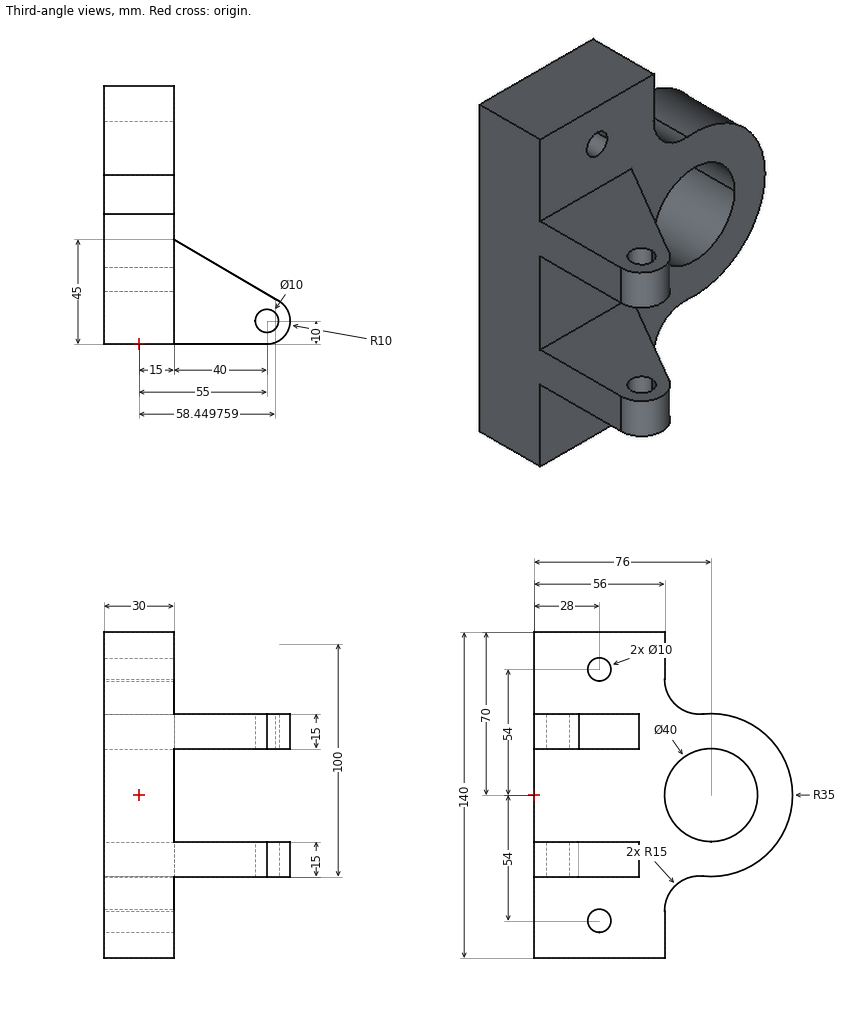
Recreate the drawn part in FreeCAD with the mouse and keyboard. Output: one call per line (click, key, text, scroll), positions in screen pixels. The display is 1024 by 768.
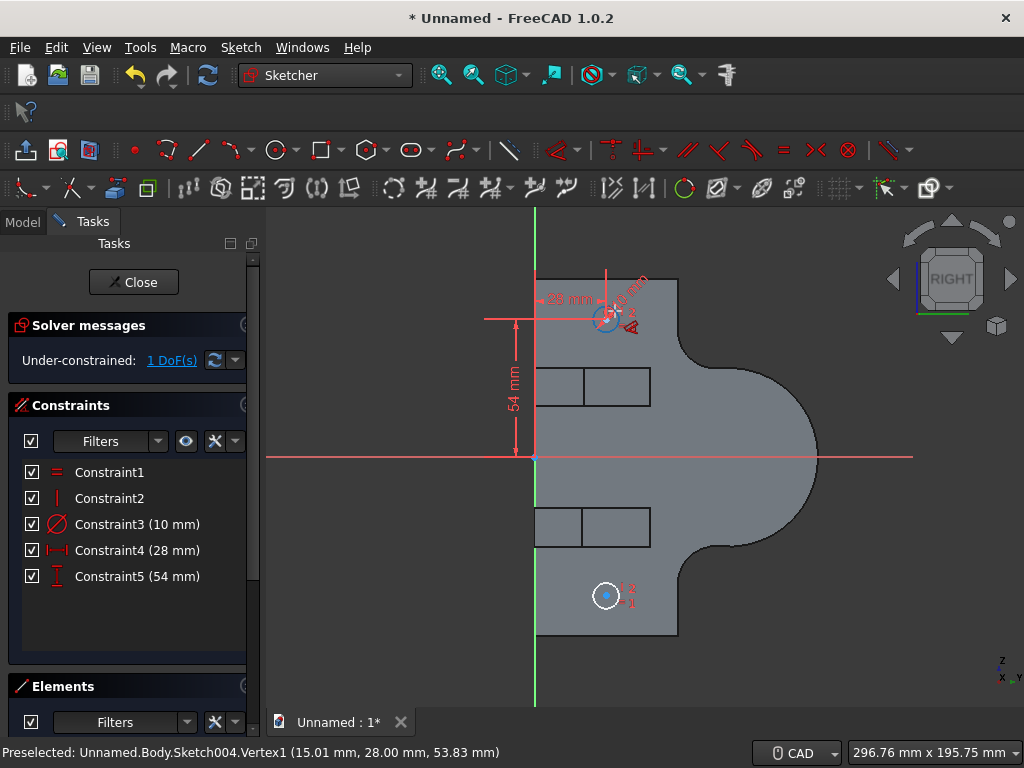
click(606, 596)
click(501, 527)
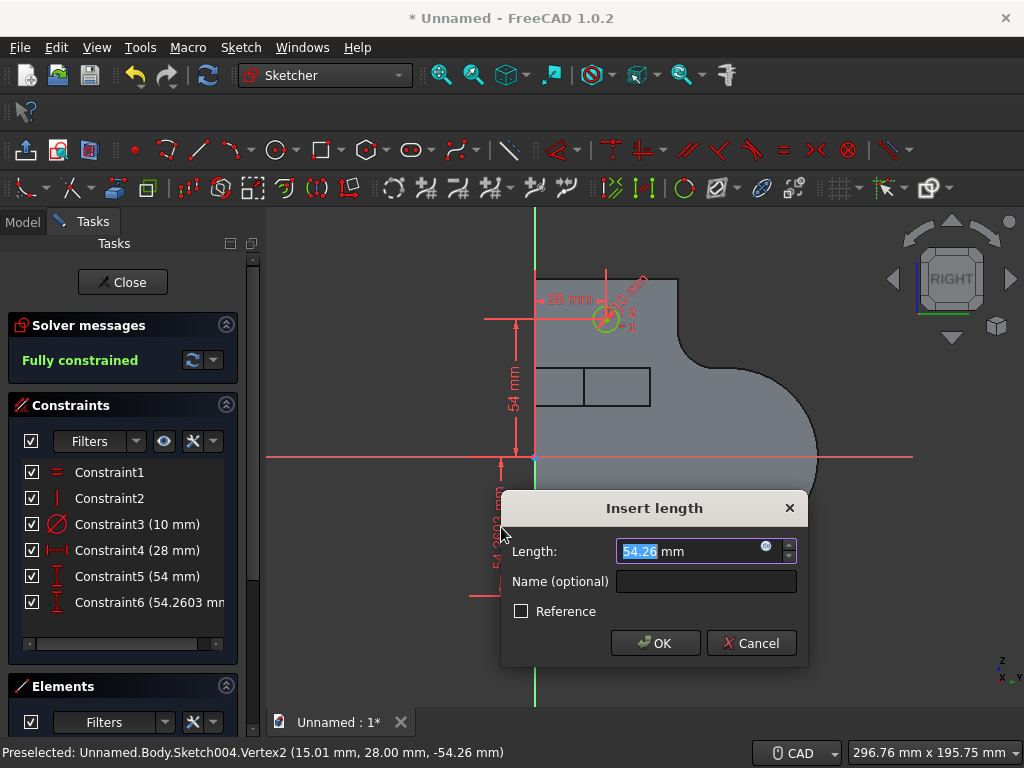
text(54)
key(Return)
key(Escape)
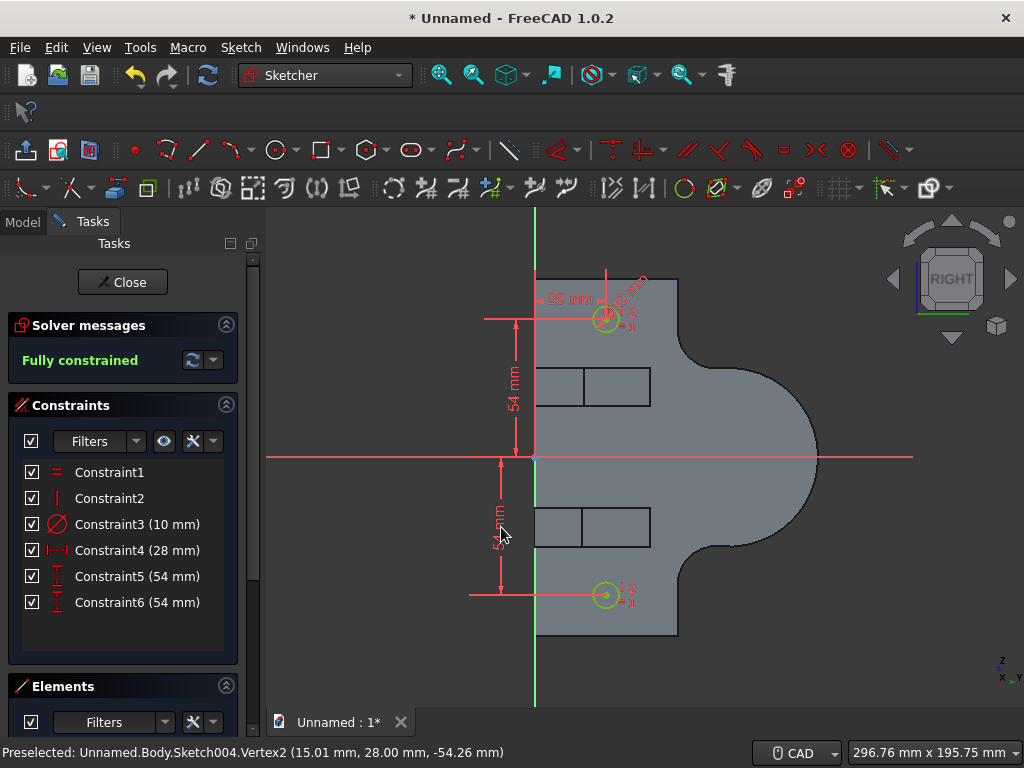
click(123, 282)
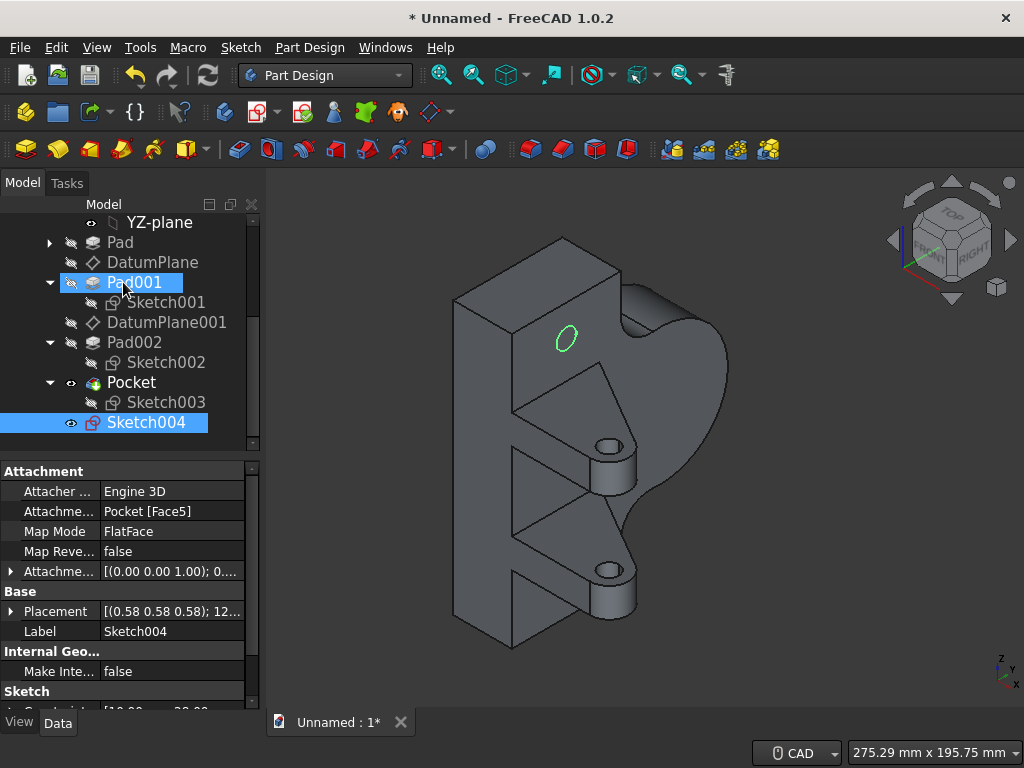
click(240, 150)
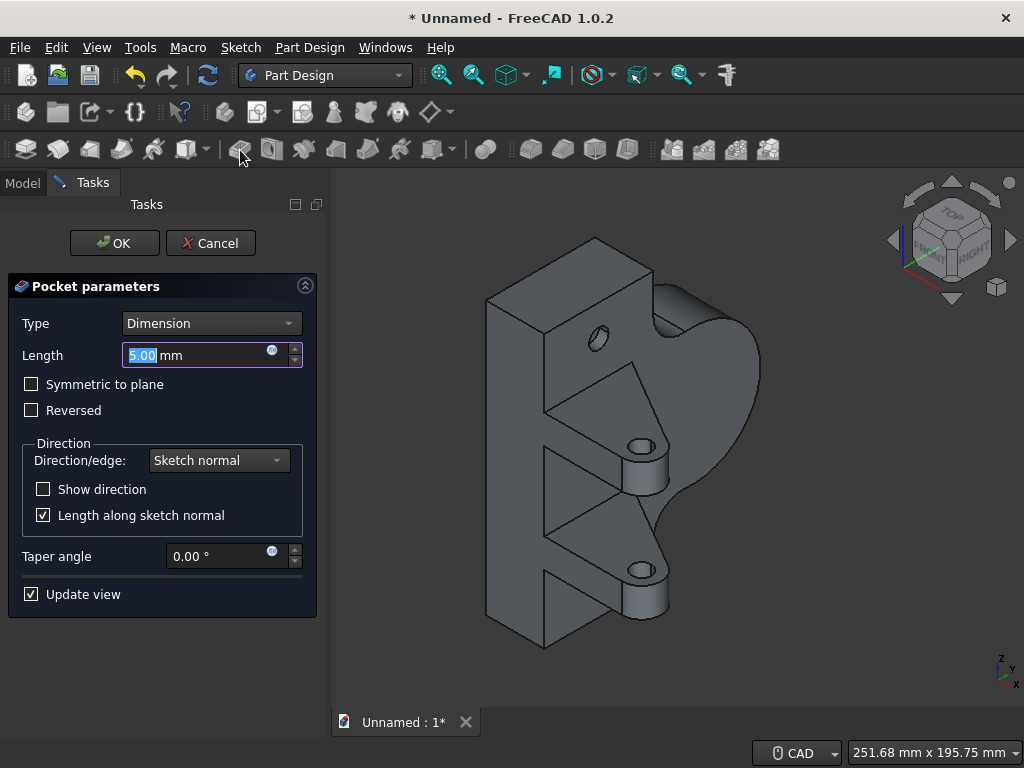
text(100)
key(Tab)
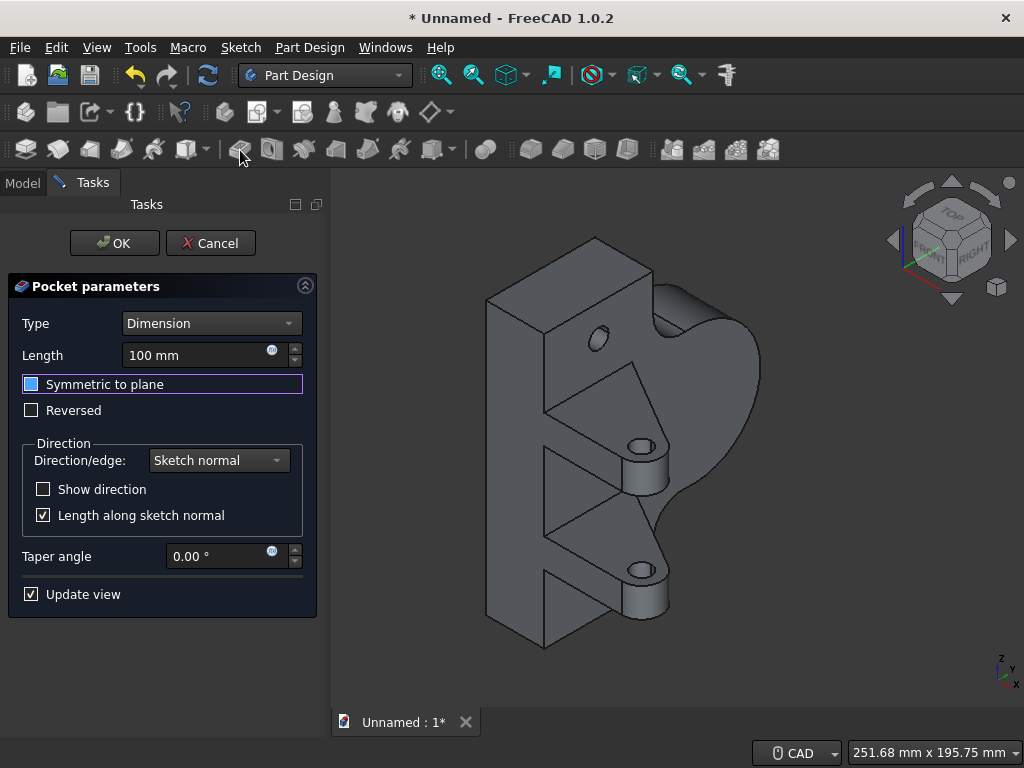
click(115, 243)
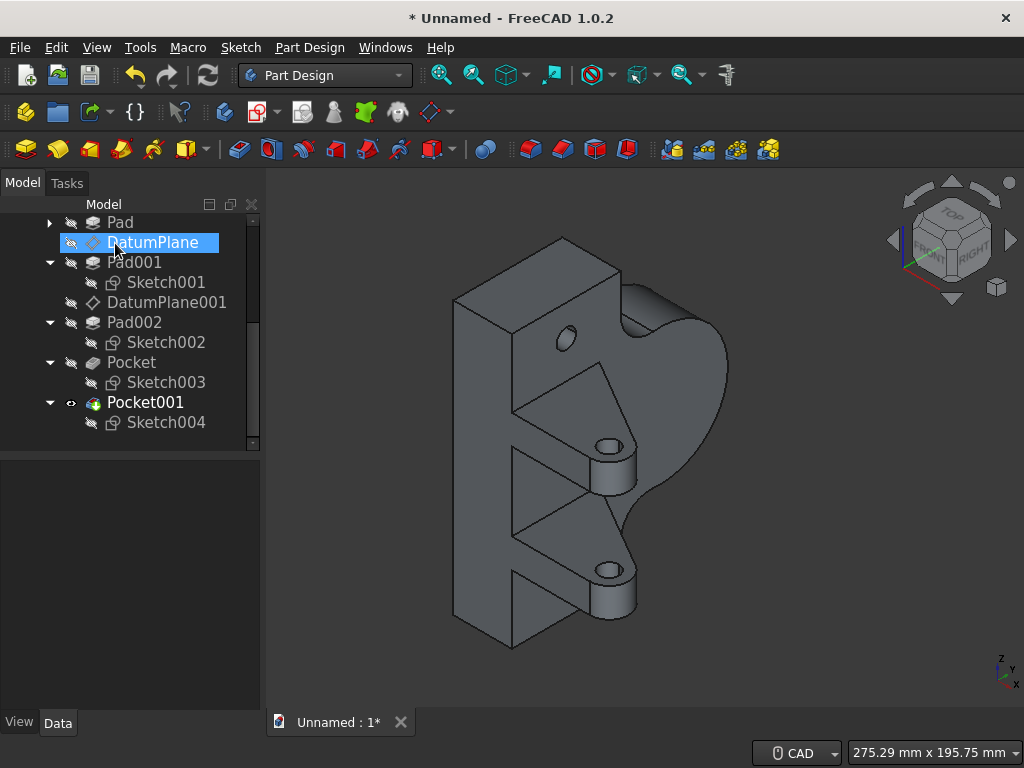
click(651, 410)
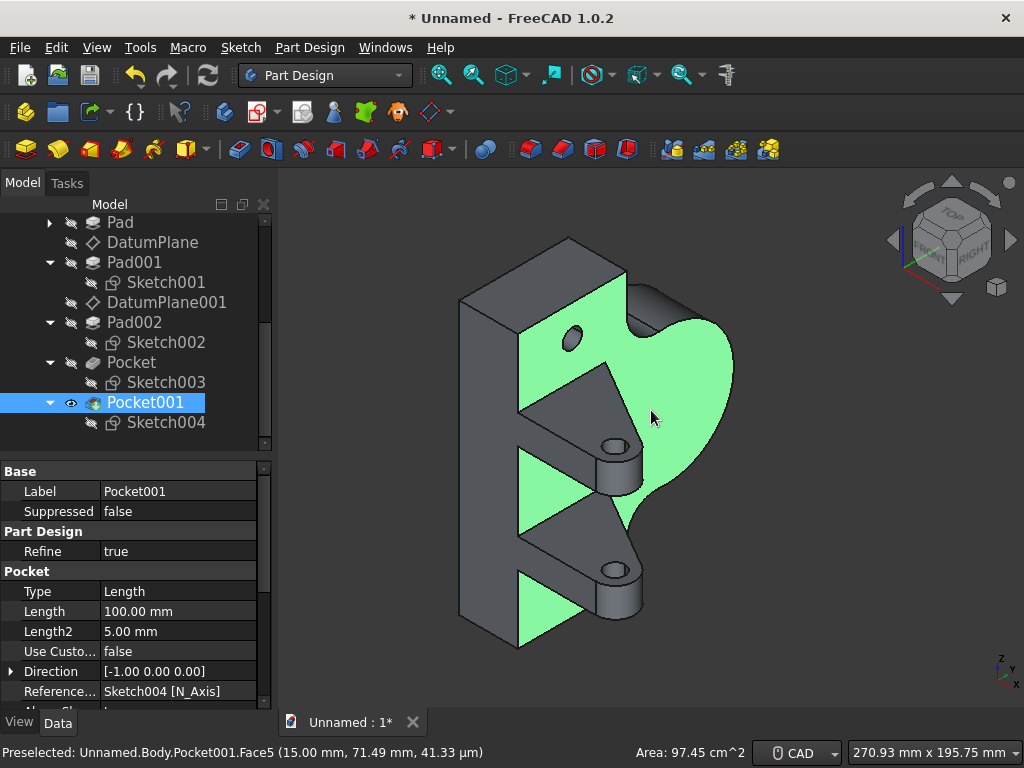
click(258, 112)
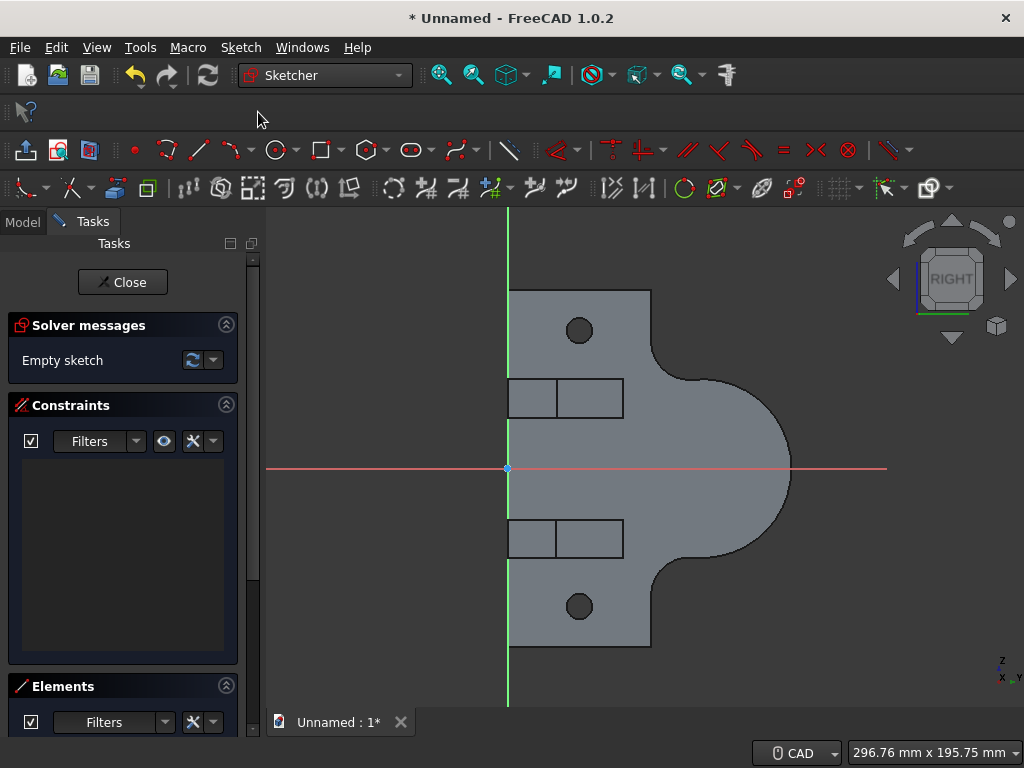
key(q)
key(s)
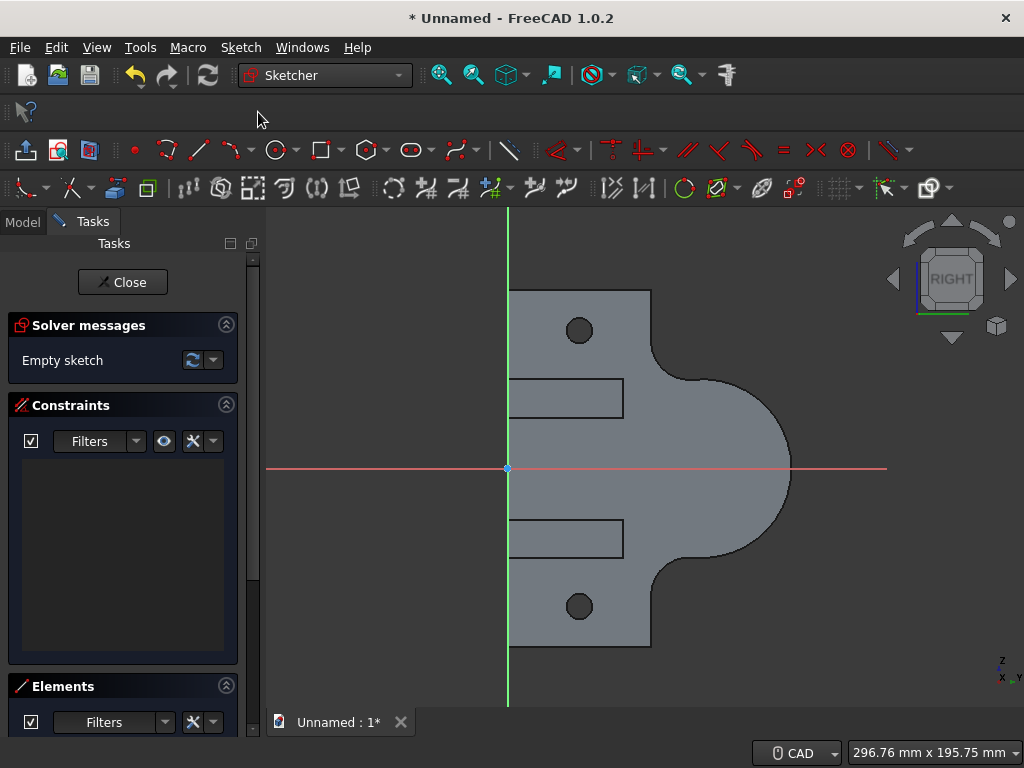
scroll(740, 492, up, 2)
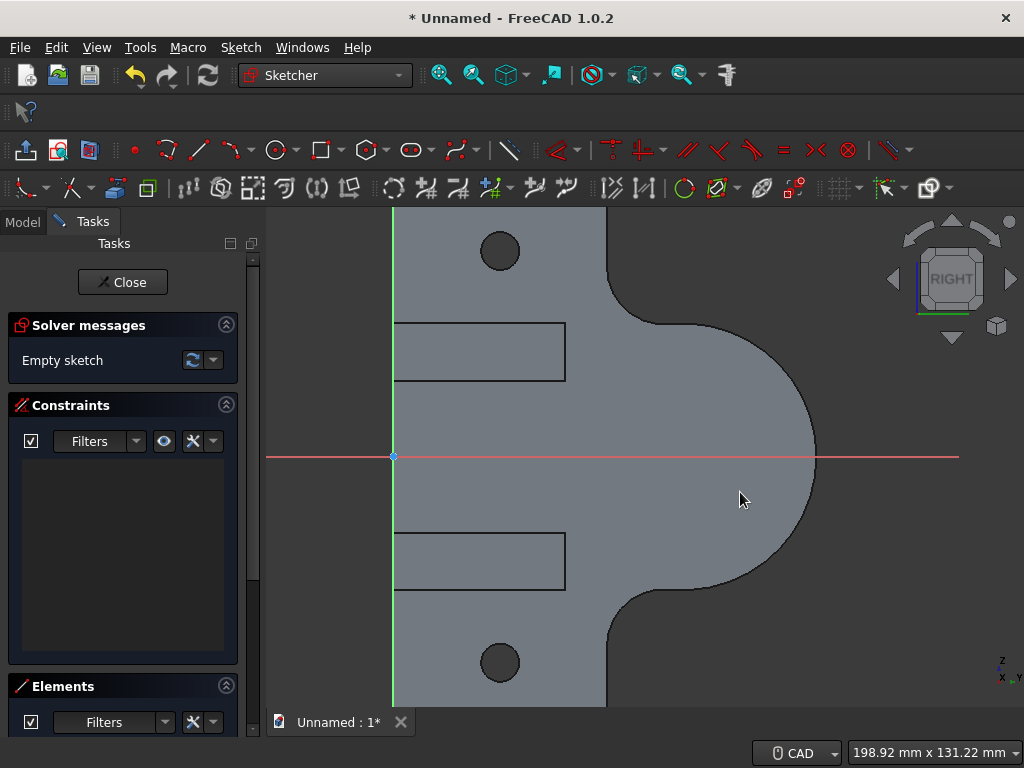
key(g)
key(c)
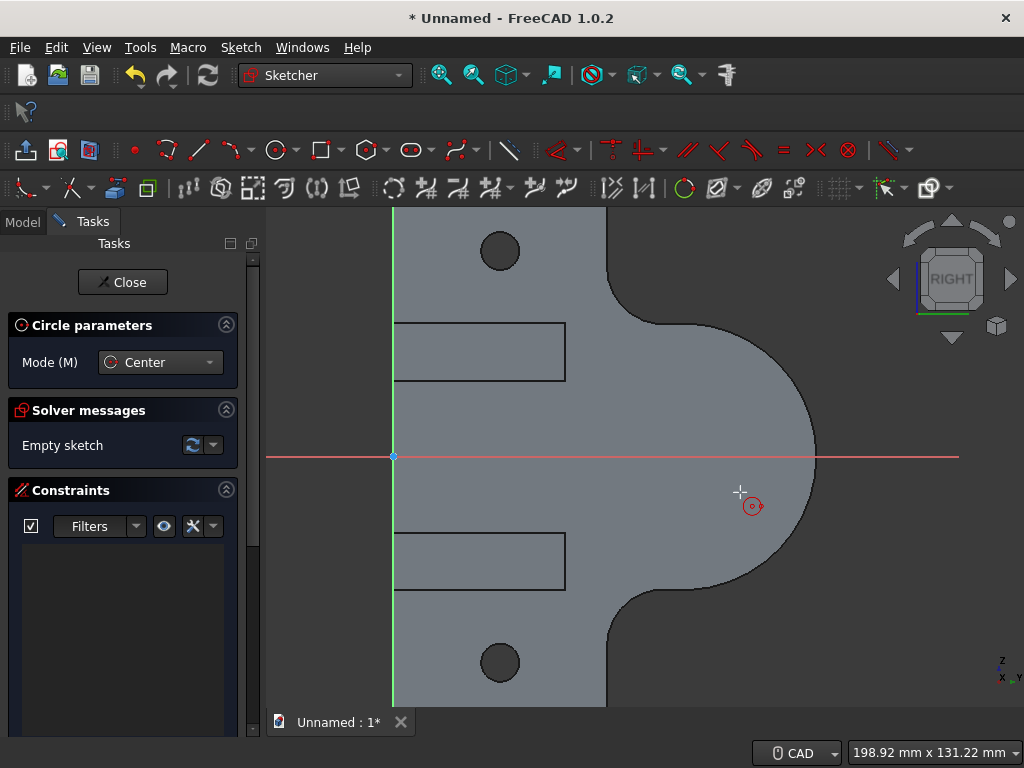
click(683, 457)
click(737, 403)
key(Escape)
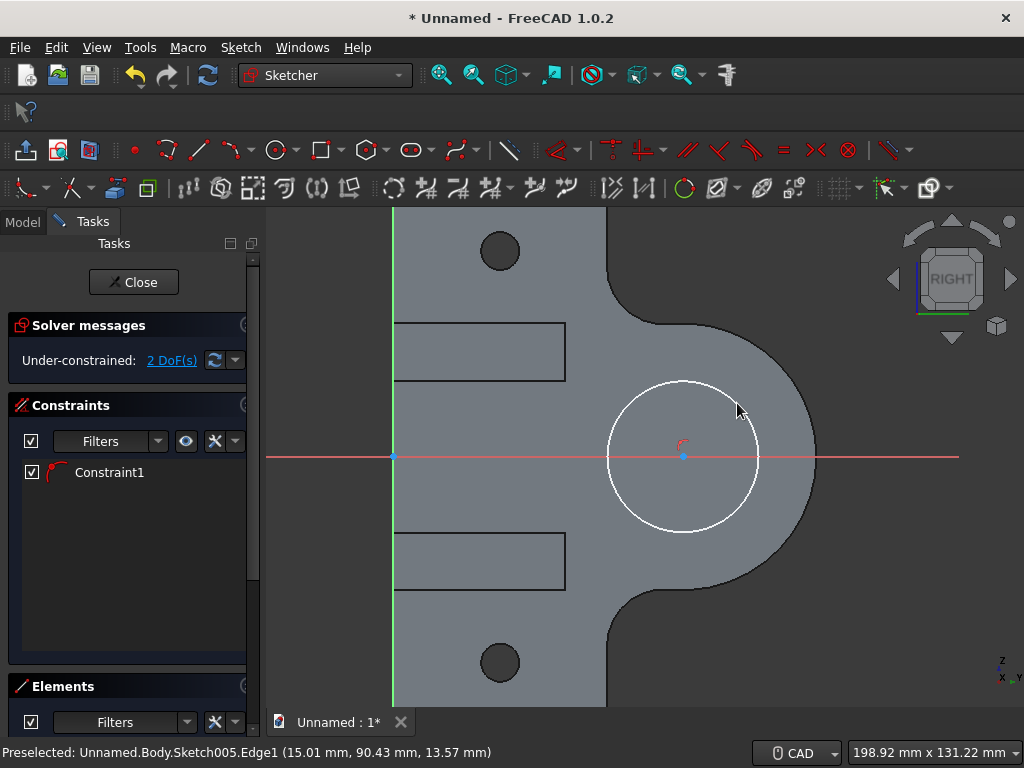
key(d)